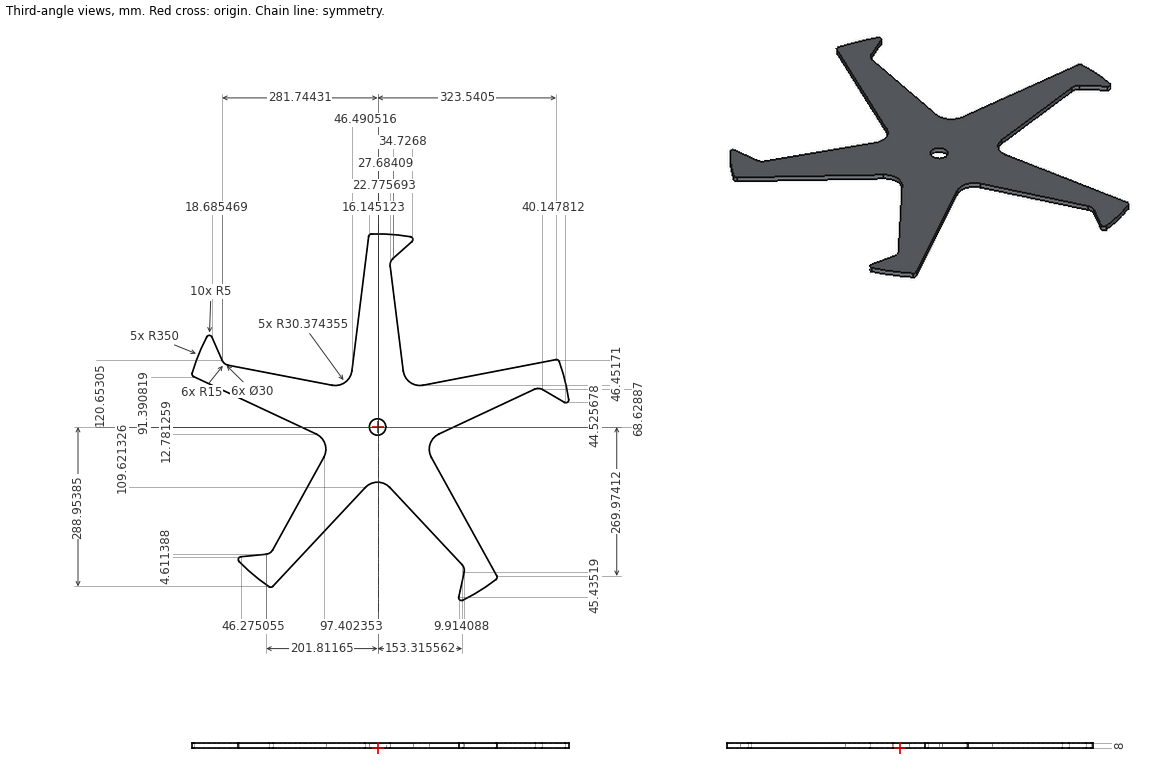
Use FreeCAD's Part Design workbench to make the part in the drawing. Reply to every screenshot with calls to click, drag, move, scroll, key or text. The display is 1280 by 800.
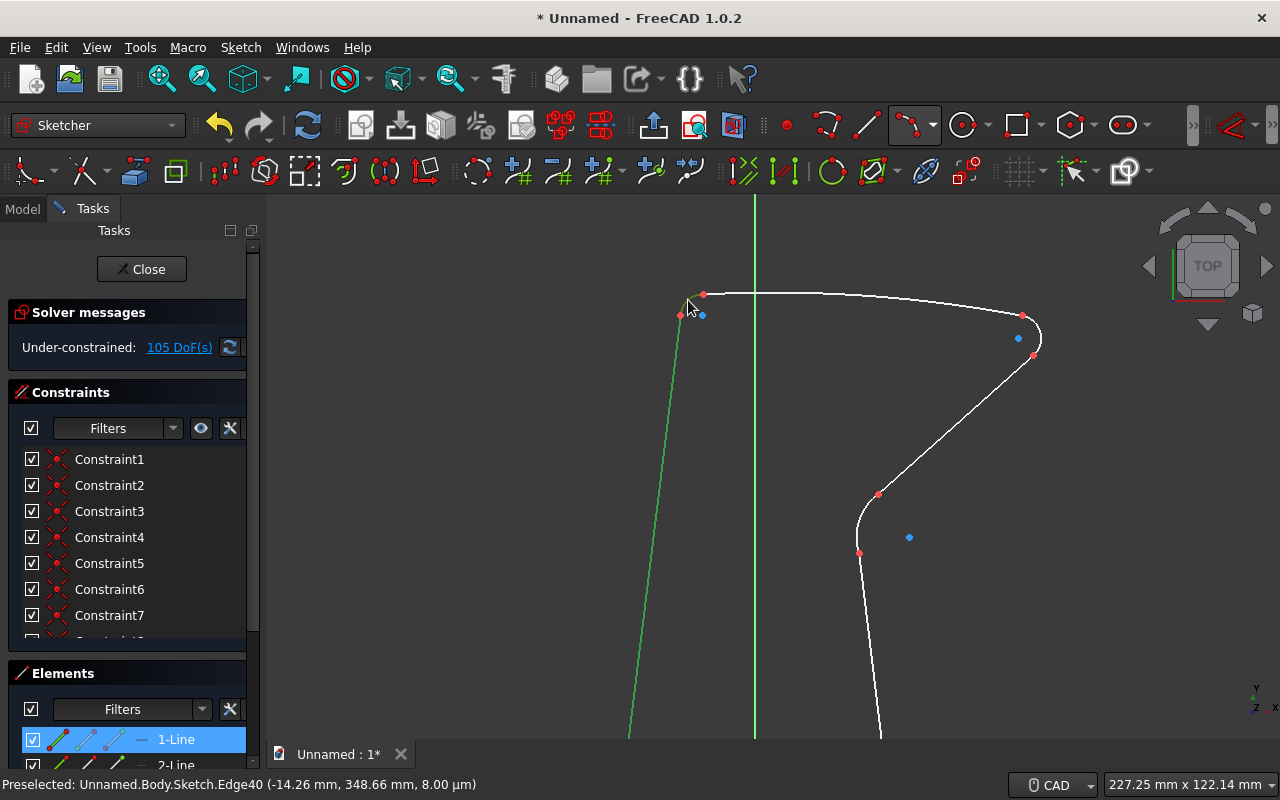
key(t)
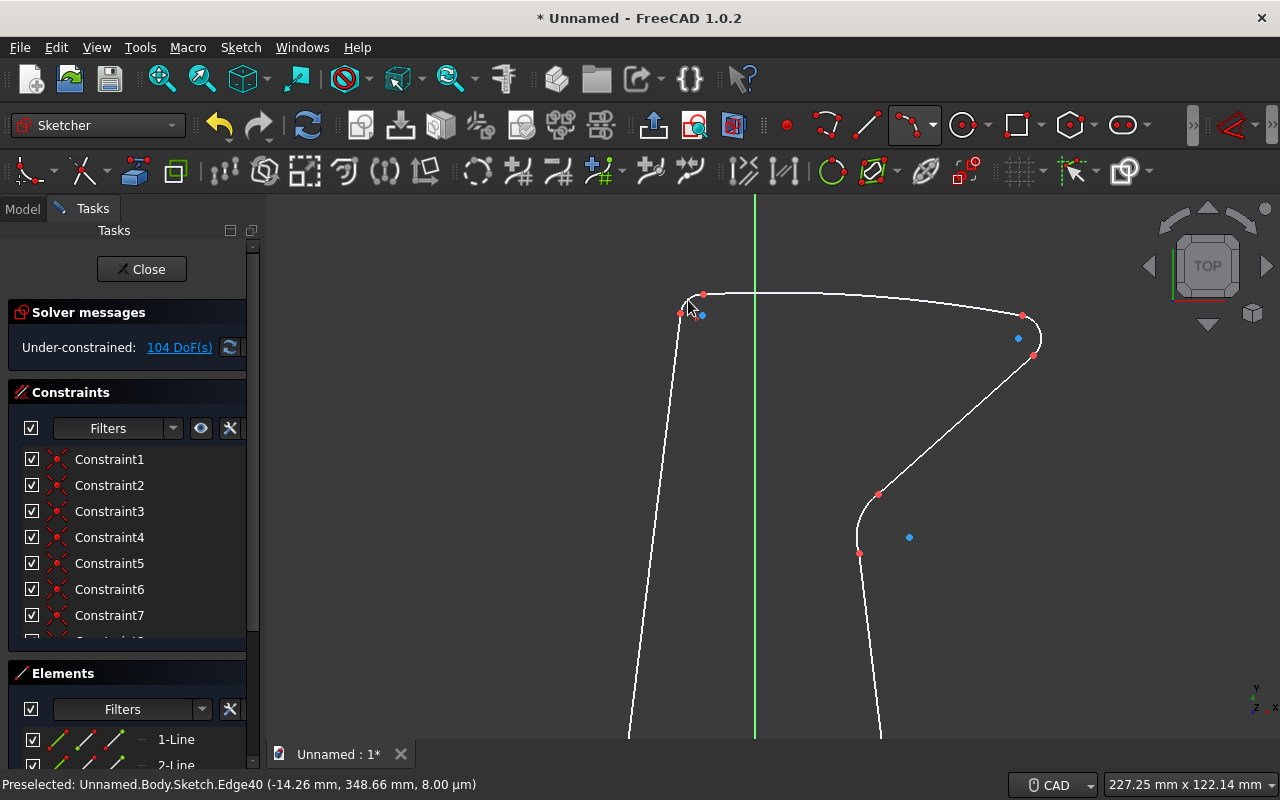
scroll(695, 304, down, 11)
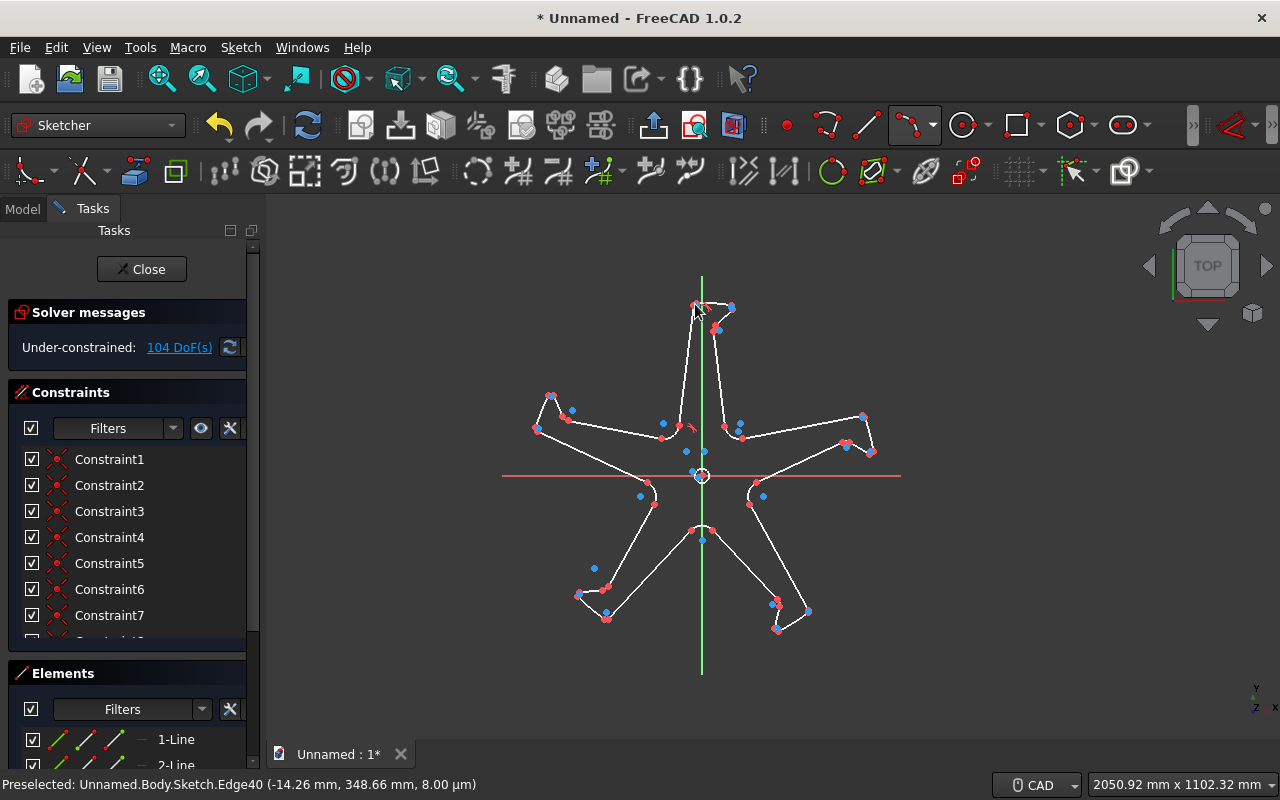
click(633, 433)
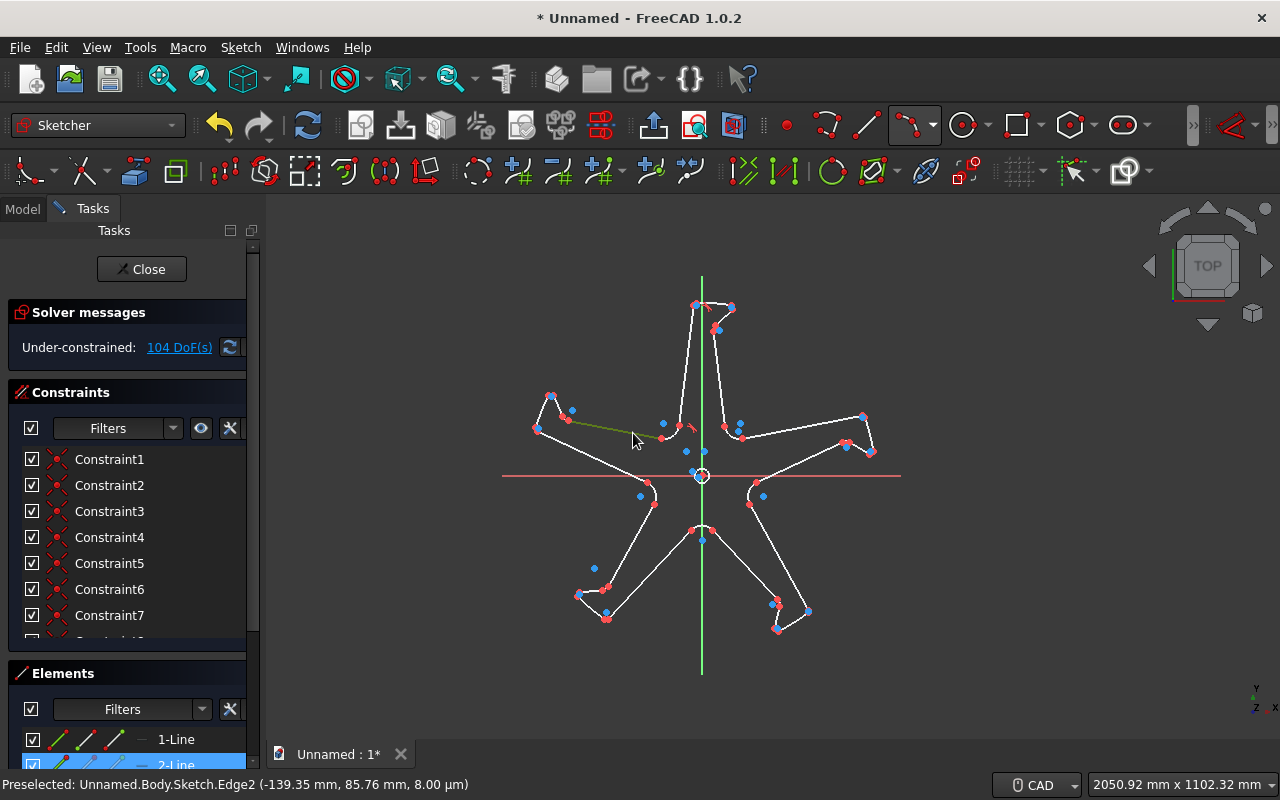
click(673, 436)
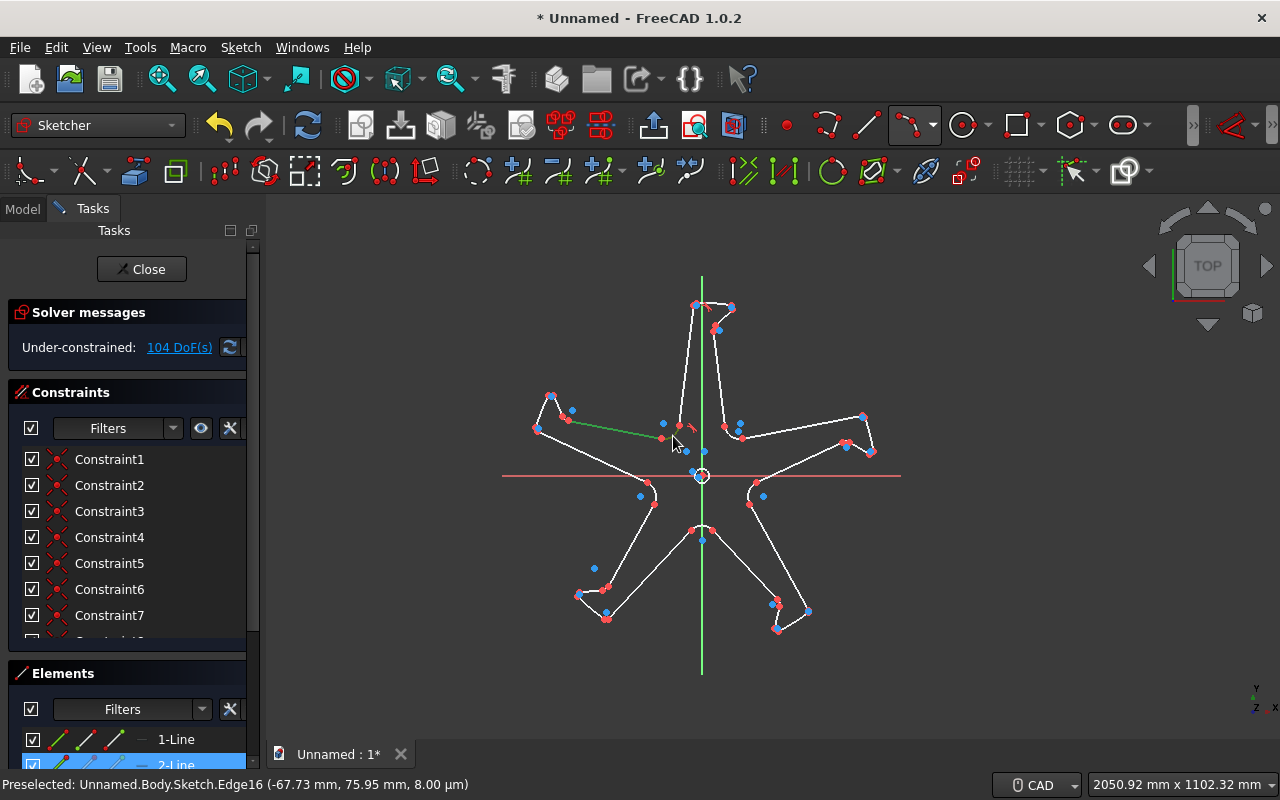
key(t)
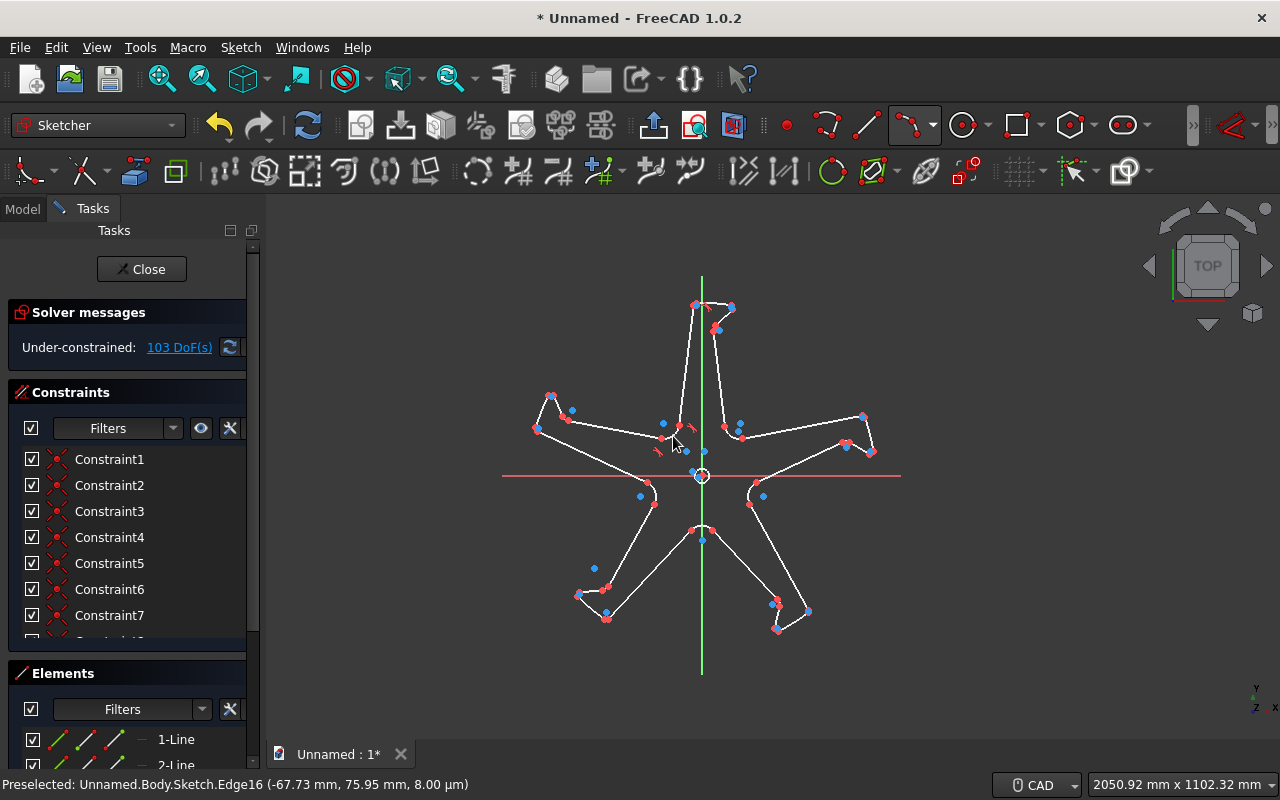
click(633, 433)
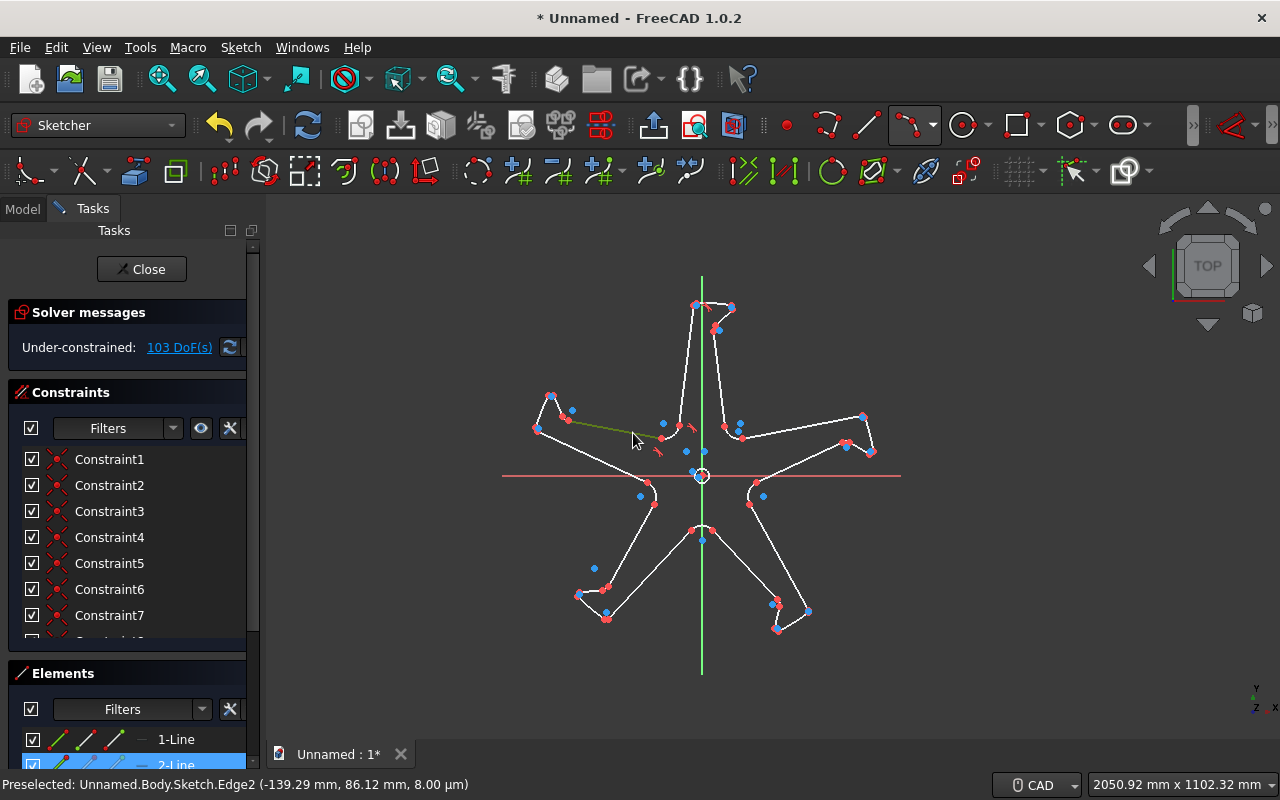
scroll(565, 419, up, 7)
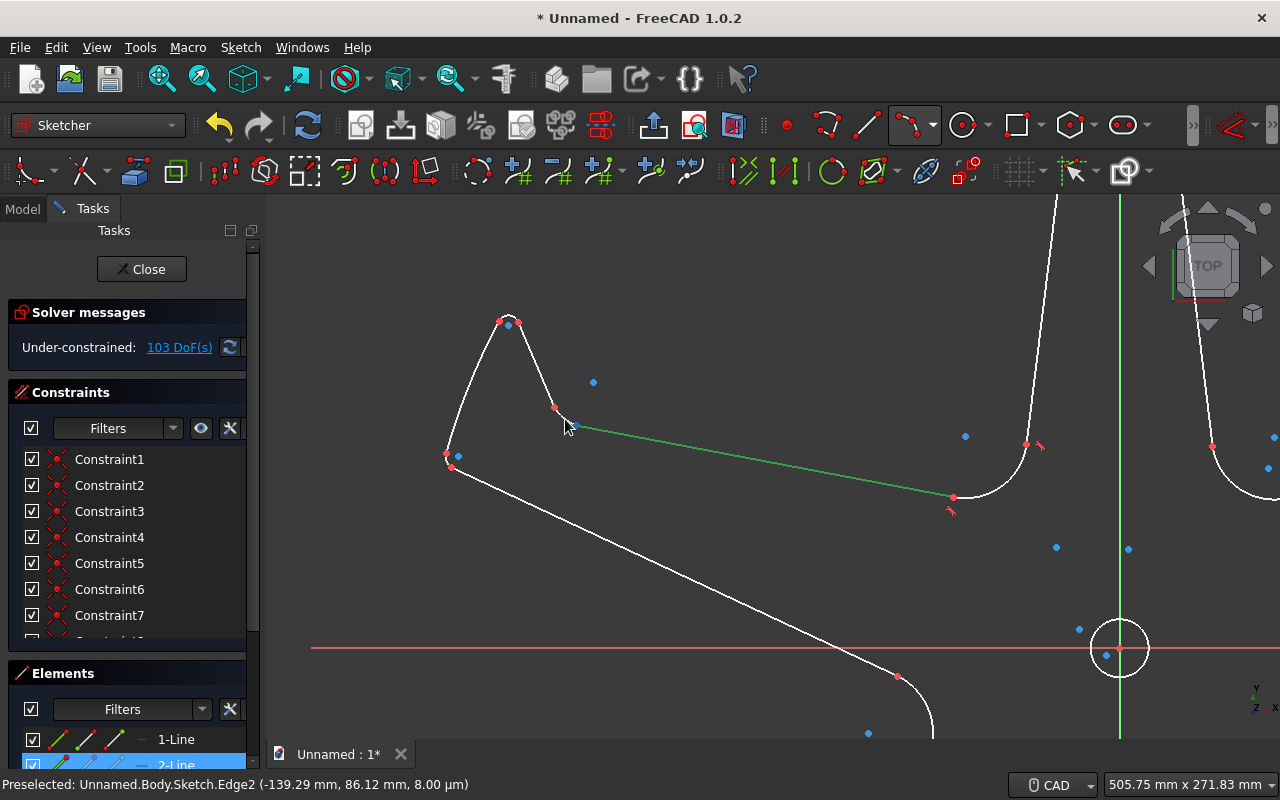
click(564, 418)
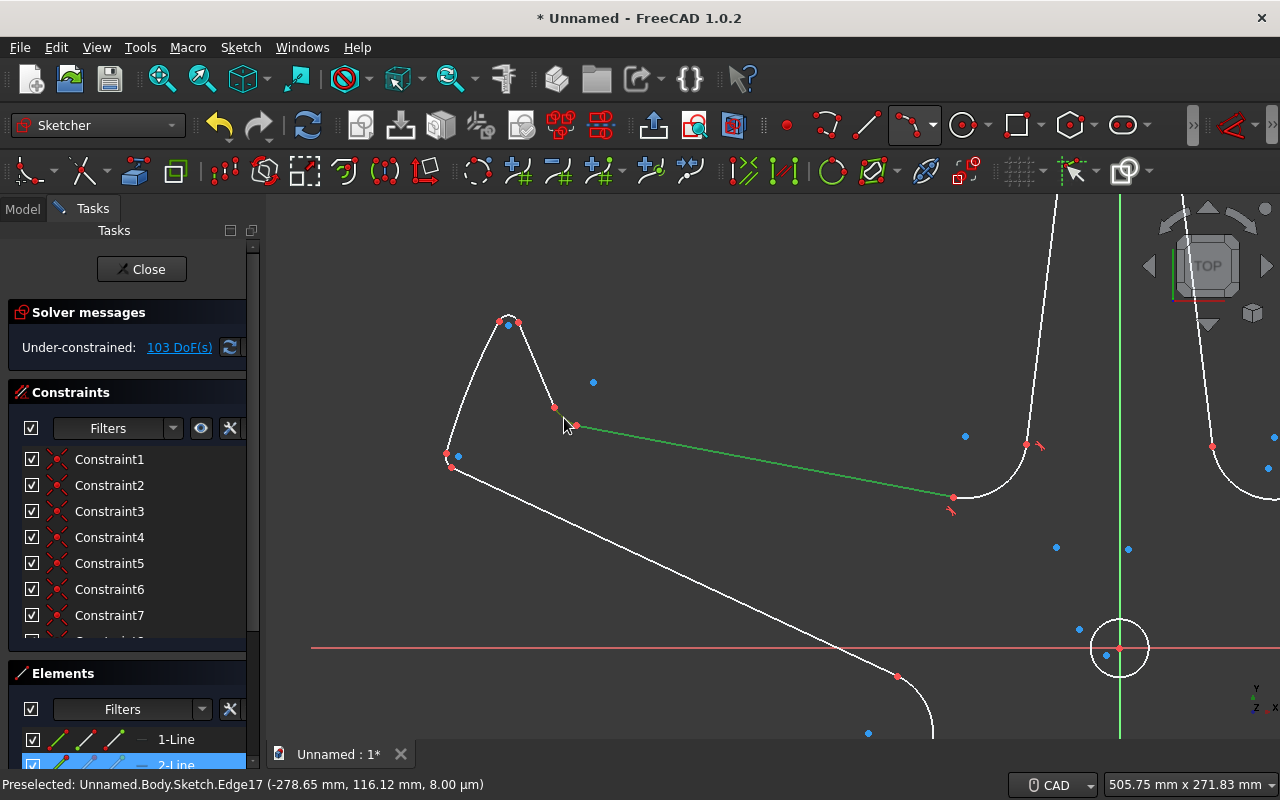
key(t)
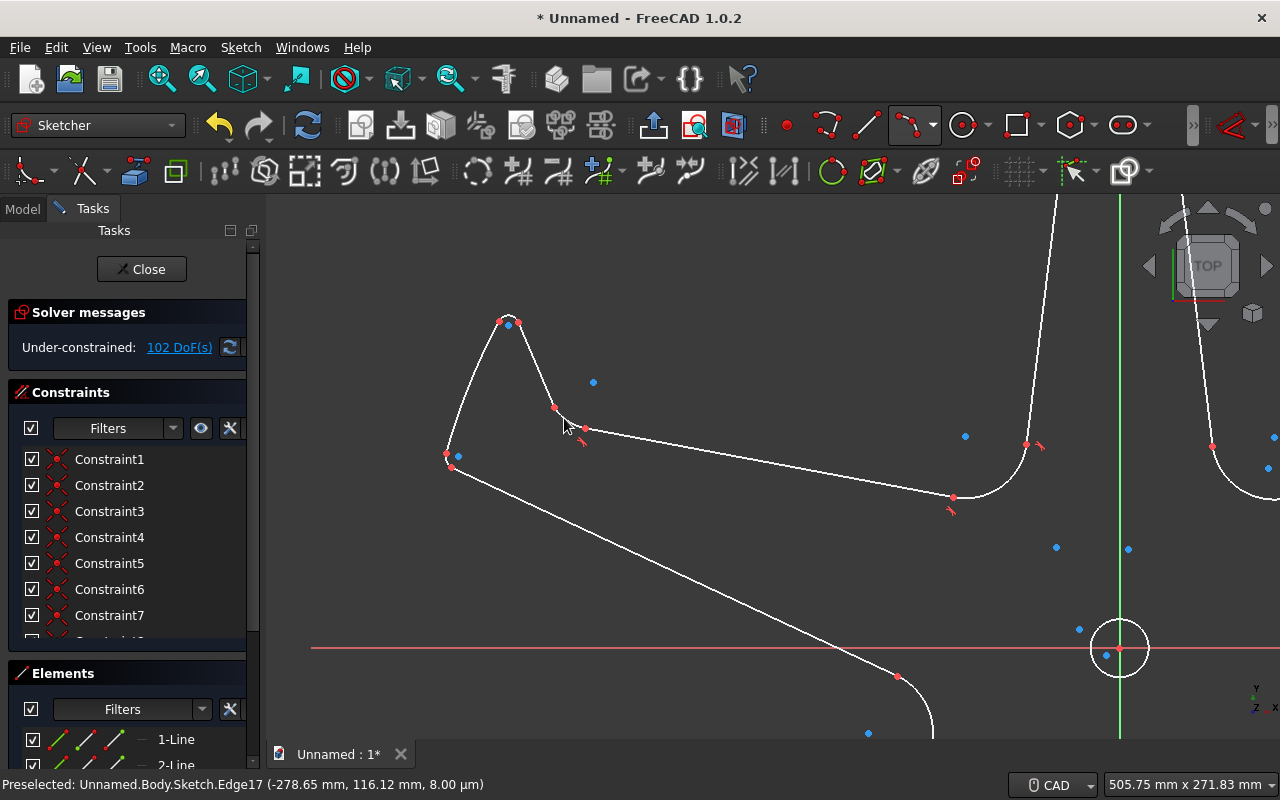
click(544, 382)